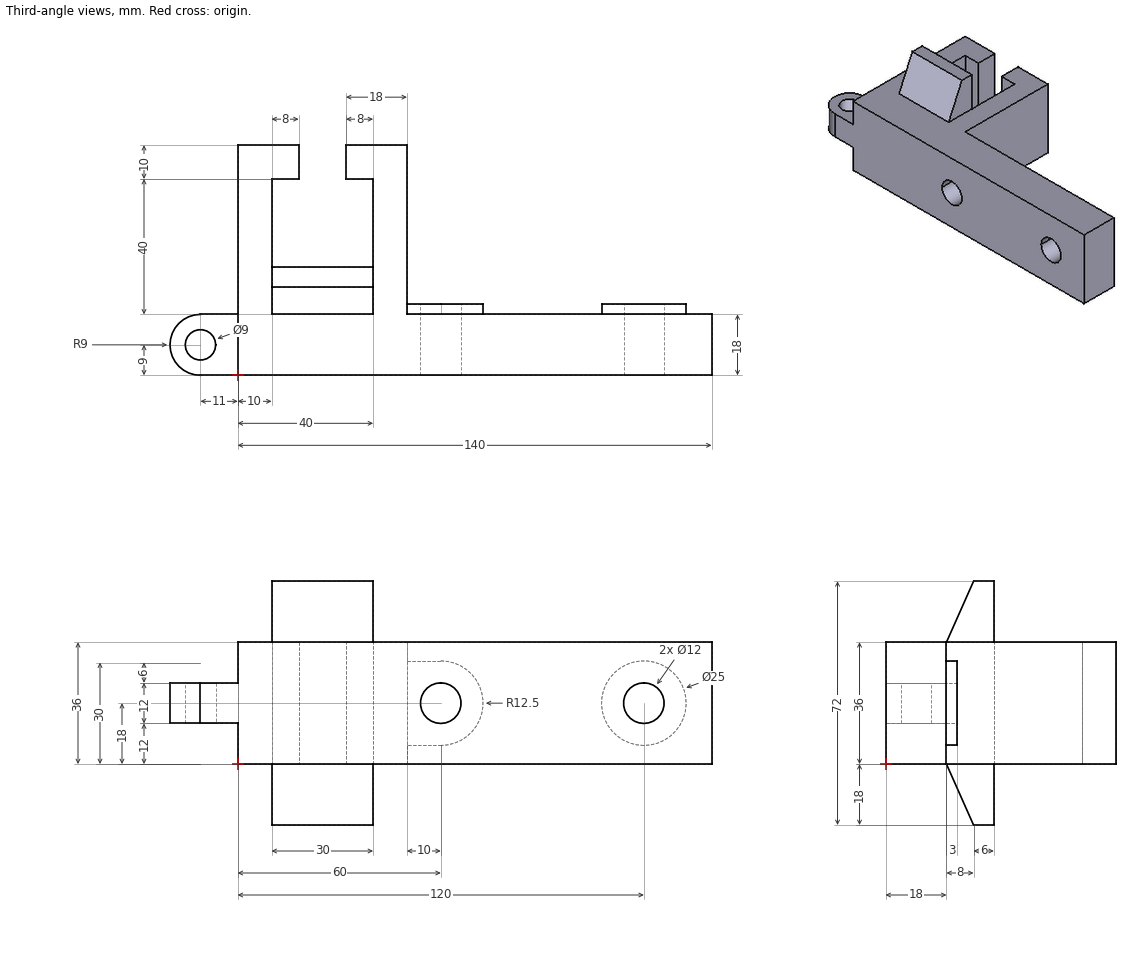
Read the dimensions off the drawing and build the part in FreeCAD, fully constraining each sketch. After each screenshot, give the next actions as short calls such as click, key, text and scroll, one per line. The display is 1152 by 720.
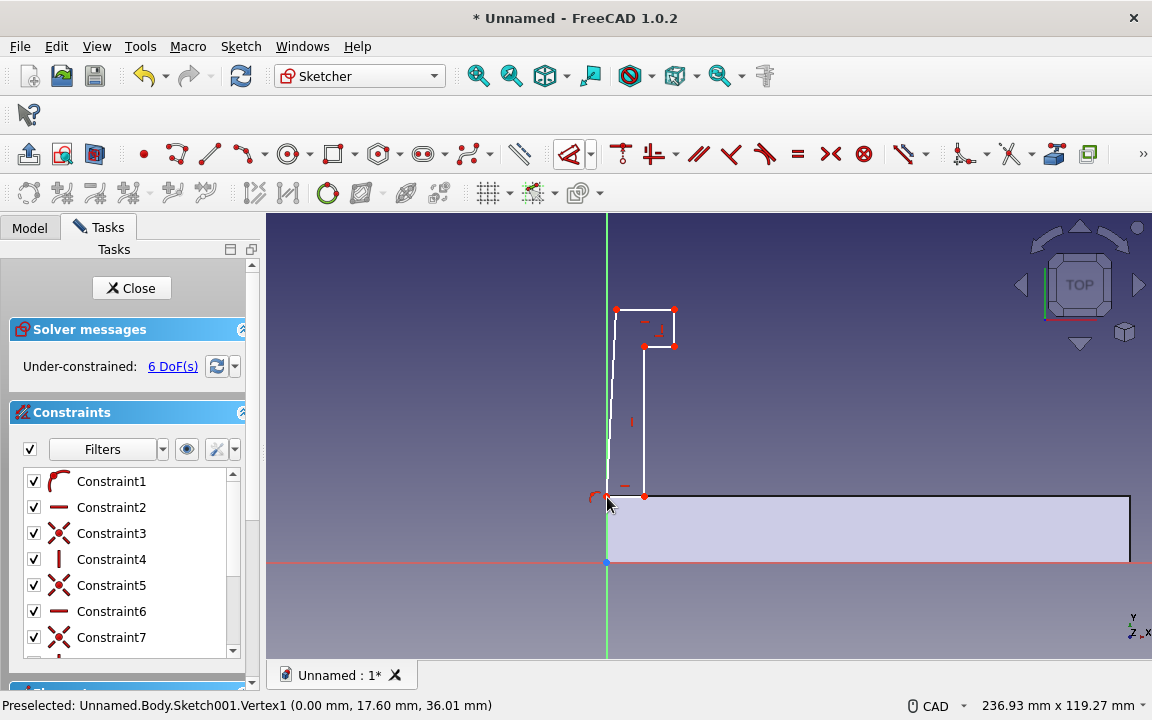
click(609, 441)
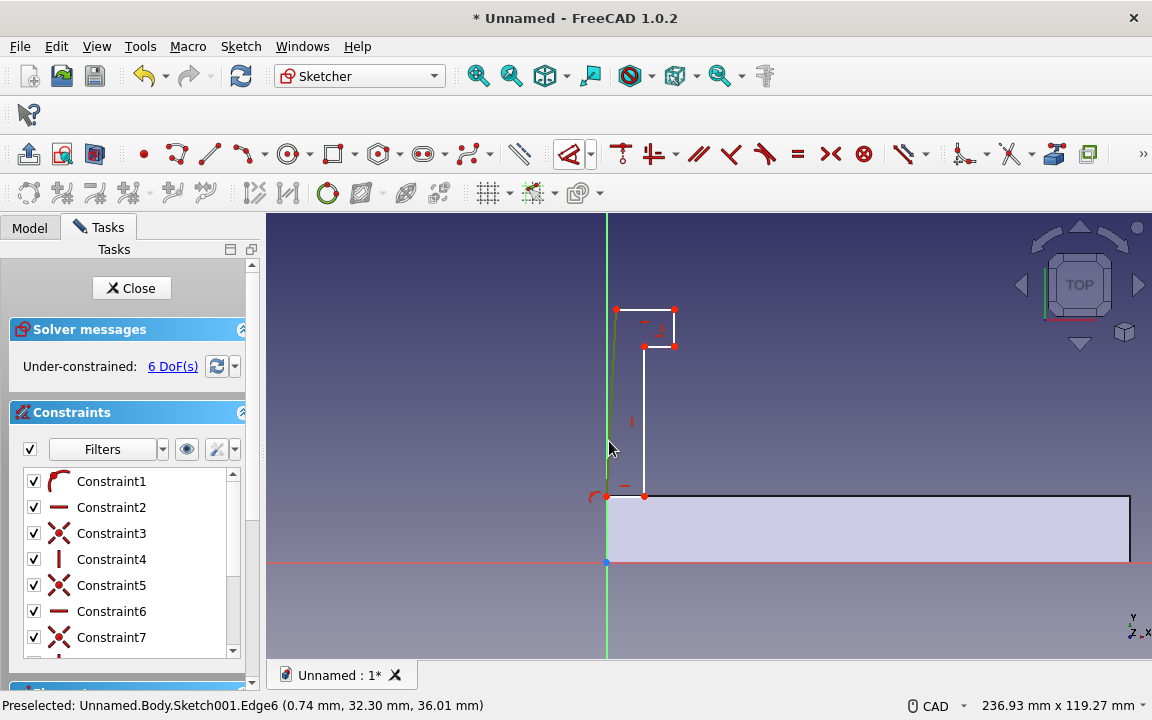
key(v)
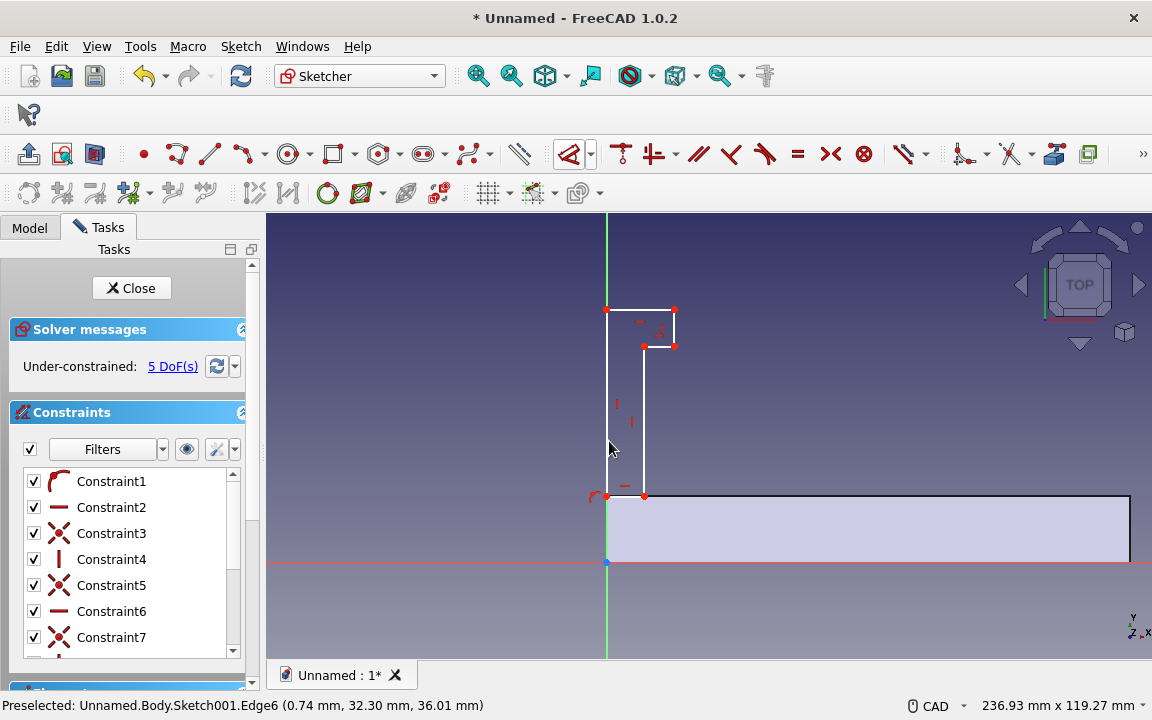
click(568, 154)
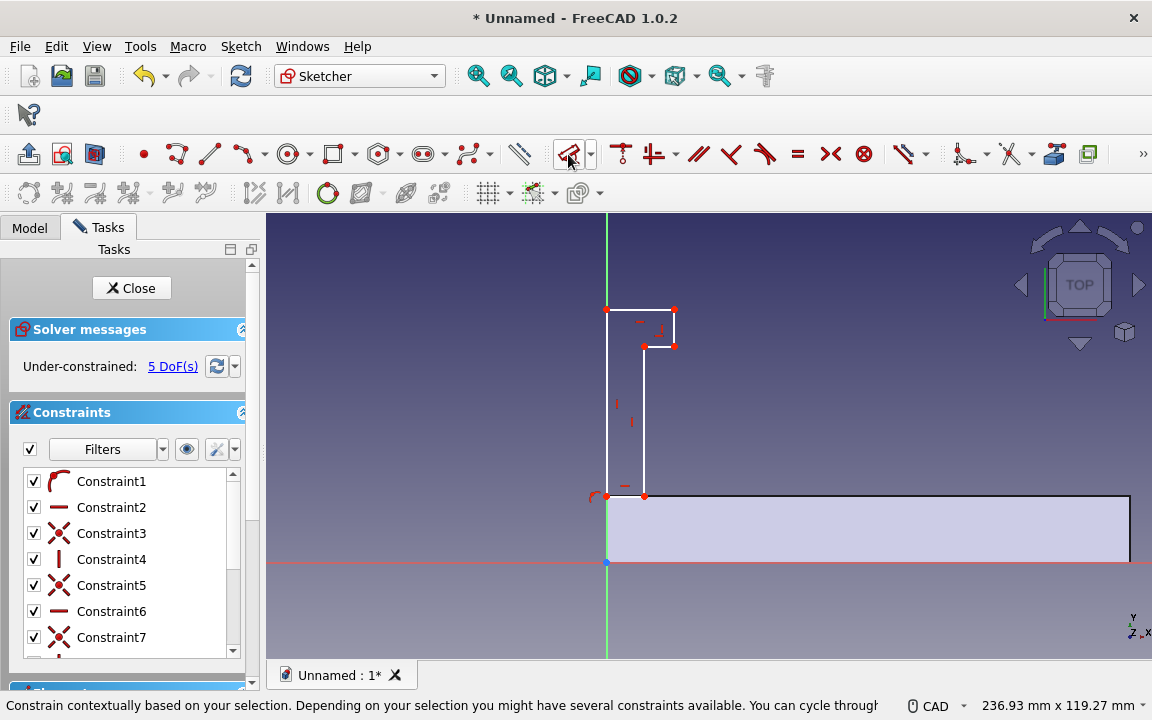
scroll(656, 347, up, 2)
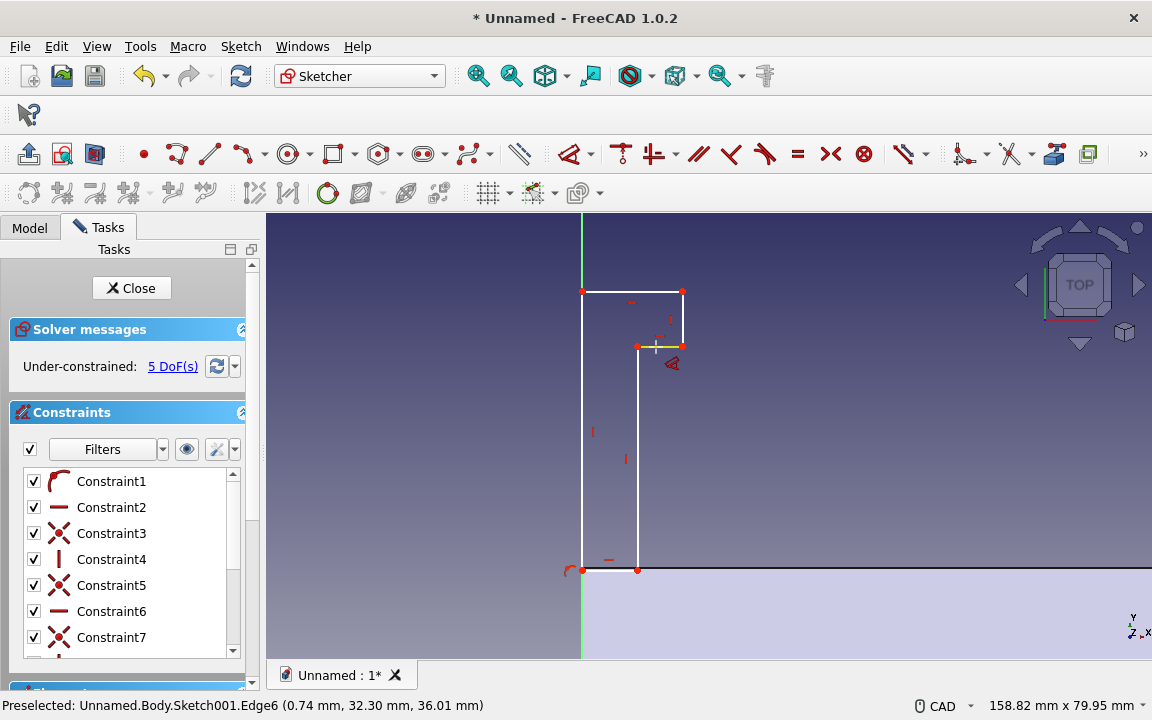
click(656, 347)
click(660, 313)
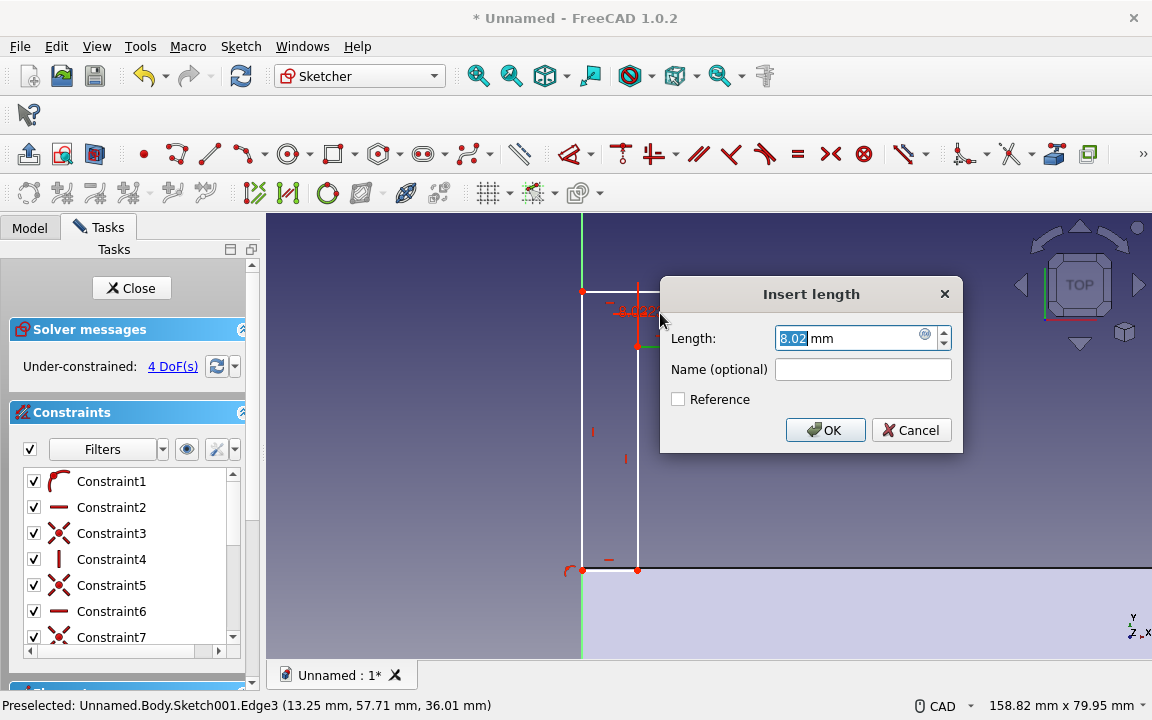
text(8)
key(Return)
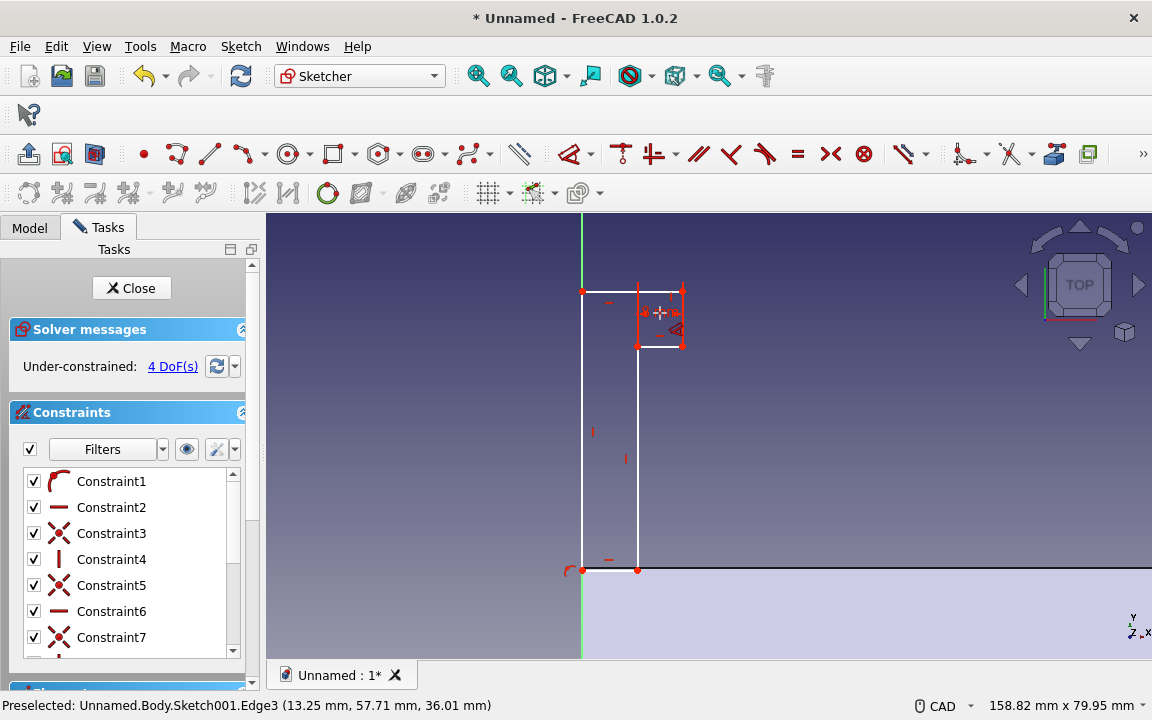
click(599, 571)
click(610, 605)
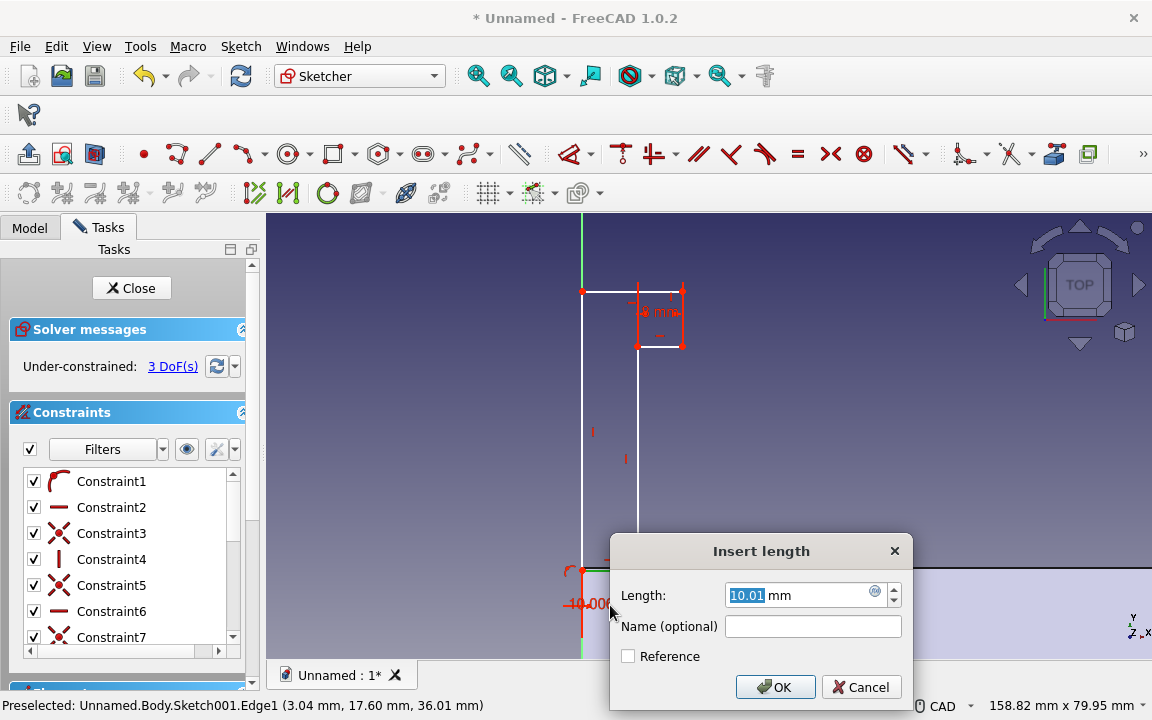
text(10)
key(Return)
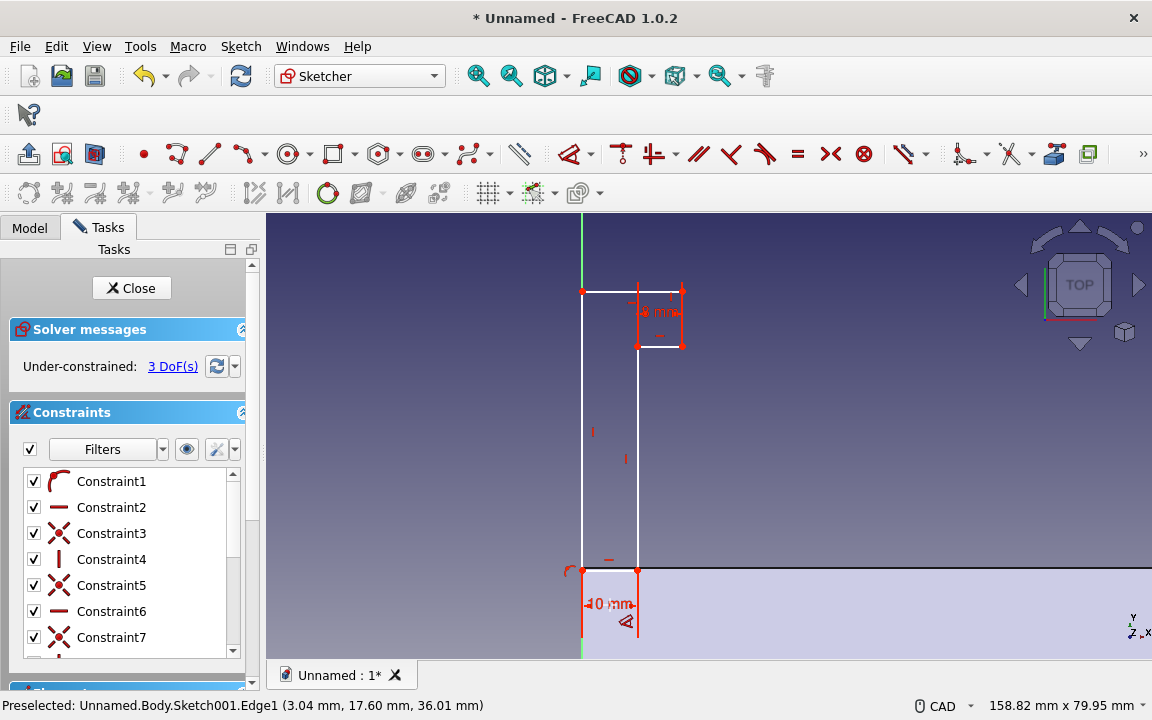
click(638, 503)
click(672, 459)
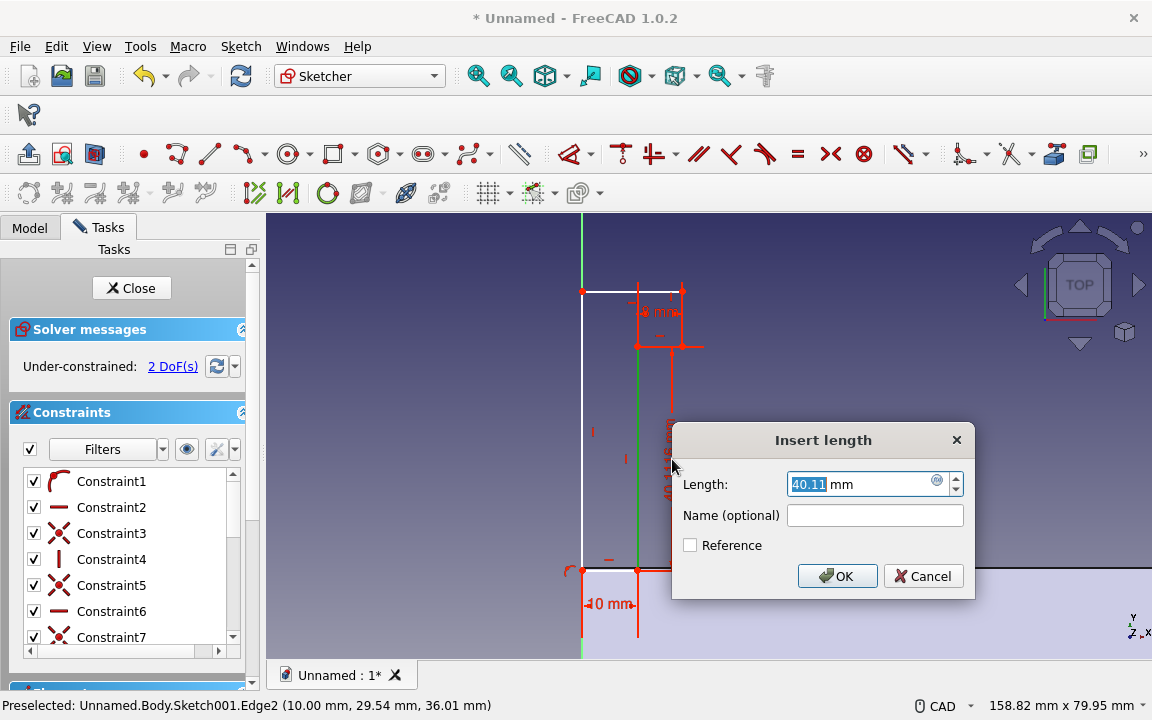
text(40)
key(Return)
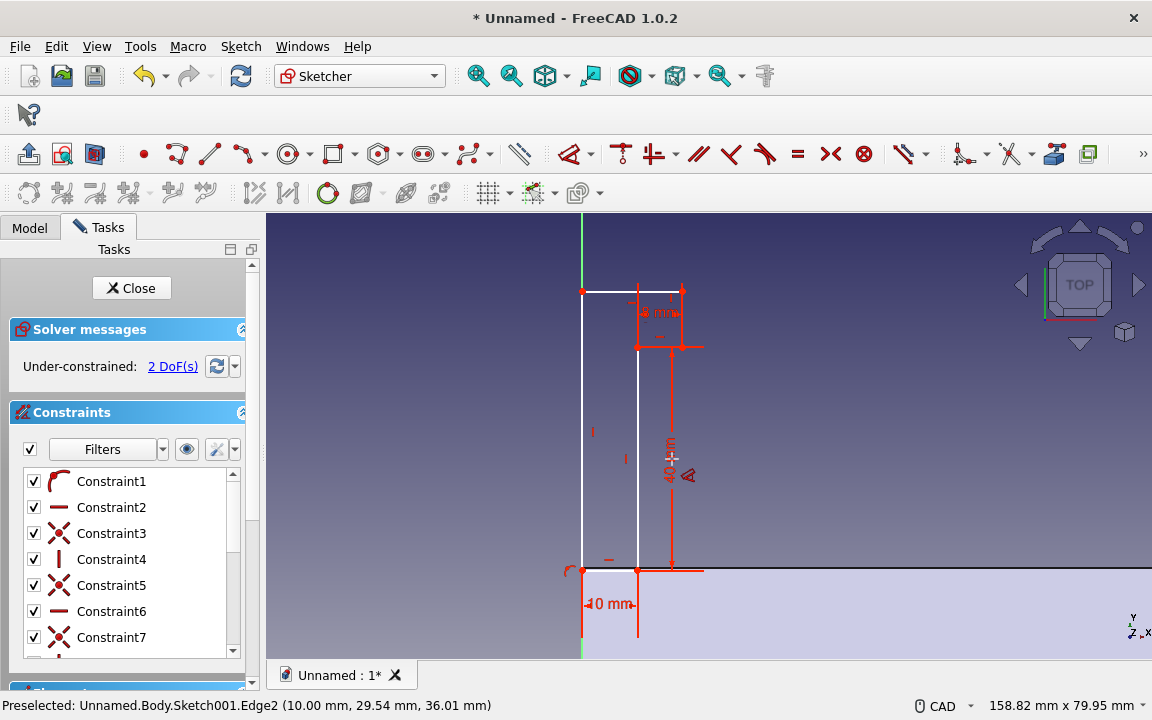
click(682, 331)
click(716, 339)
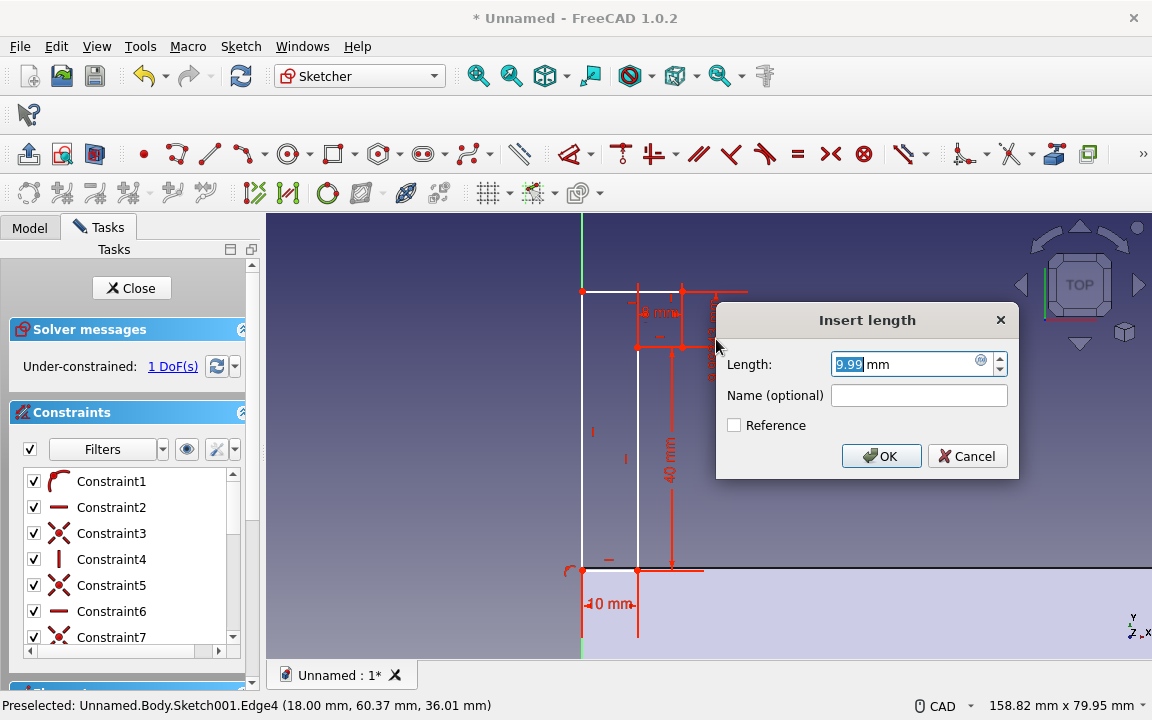
text(10)
key(Return)